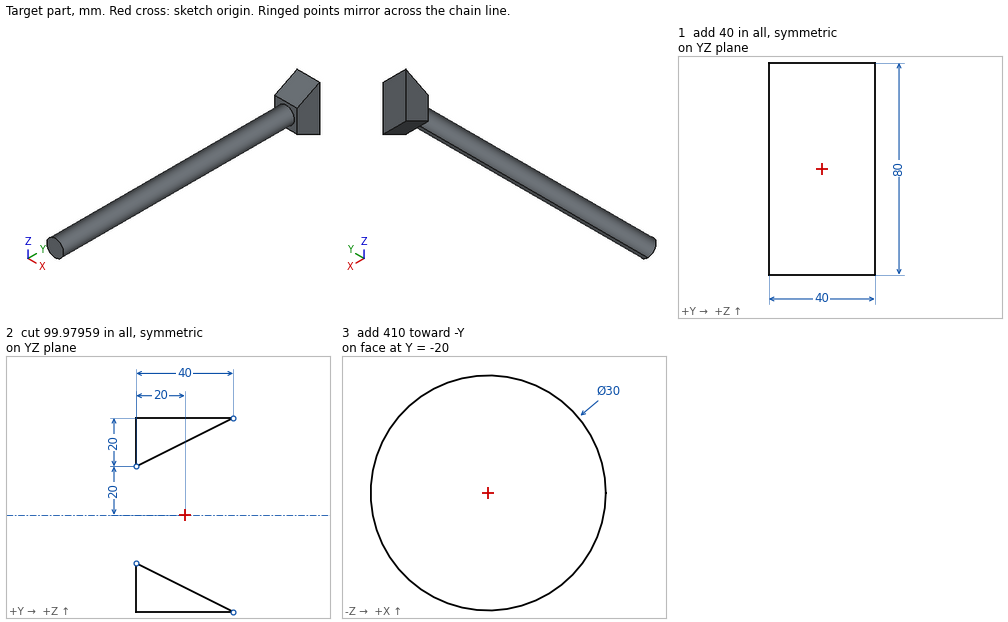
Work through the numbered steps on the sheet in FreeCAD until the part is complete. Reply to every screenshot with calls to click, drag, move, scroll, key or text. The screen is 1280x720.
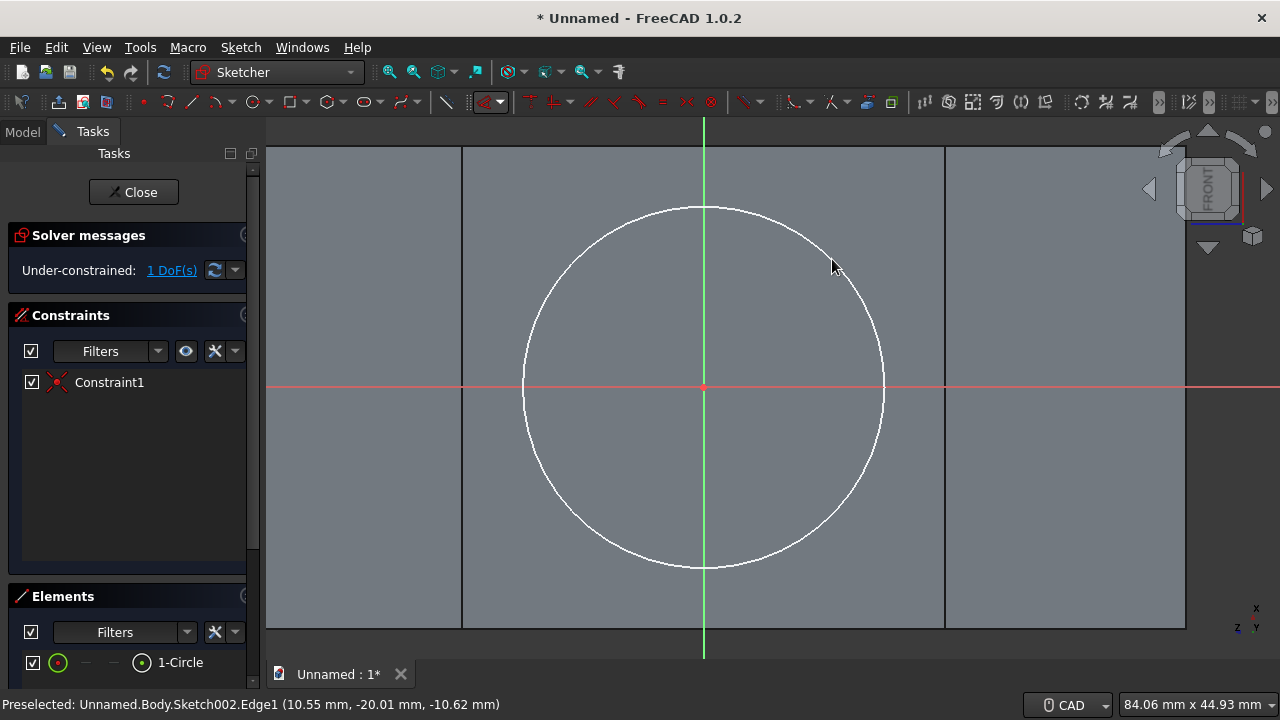
click(831, 259)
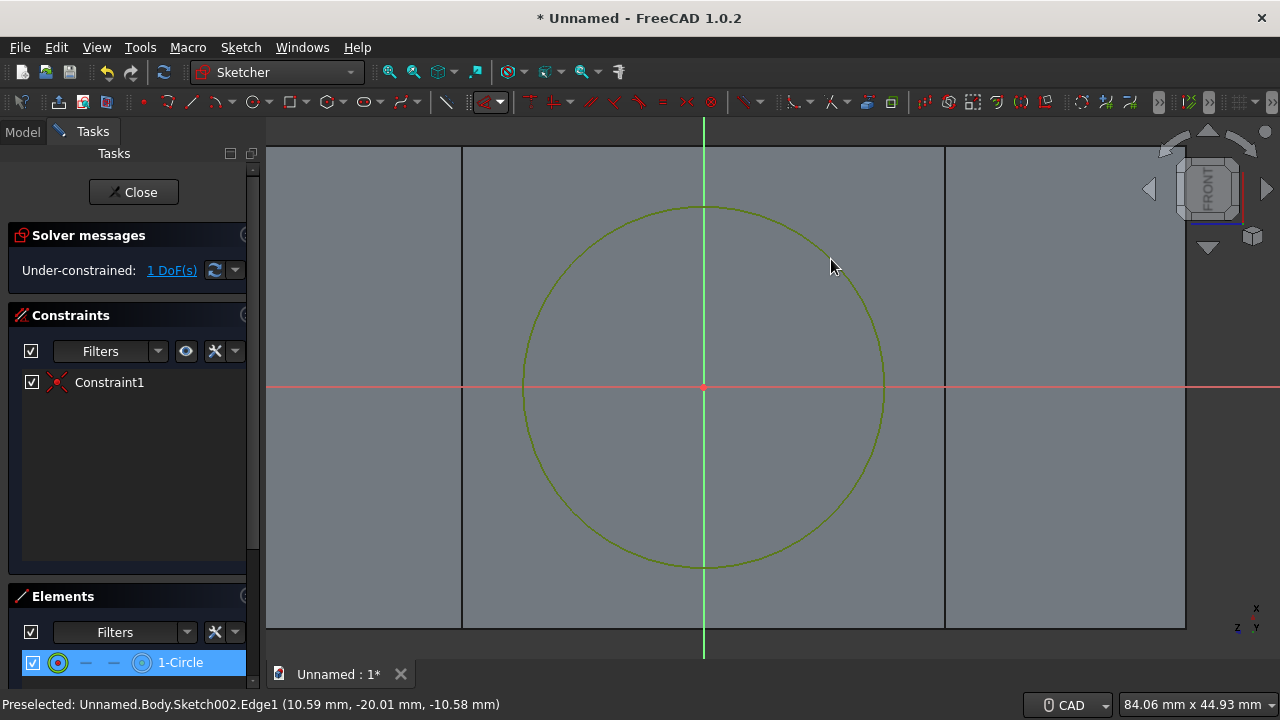
key(k)
key(o)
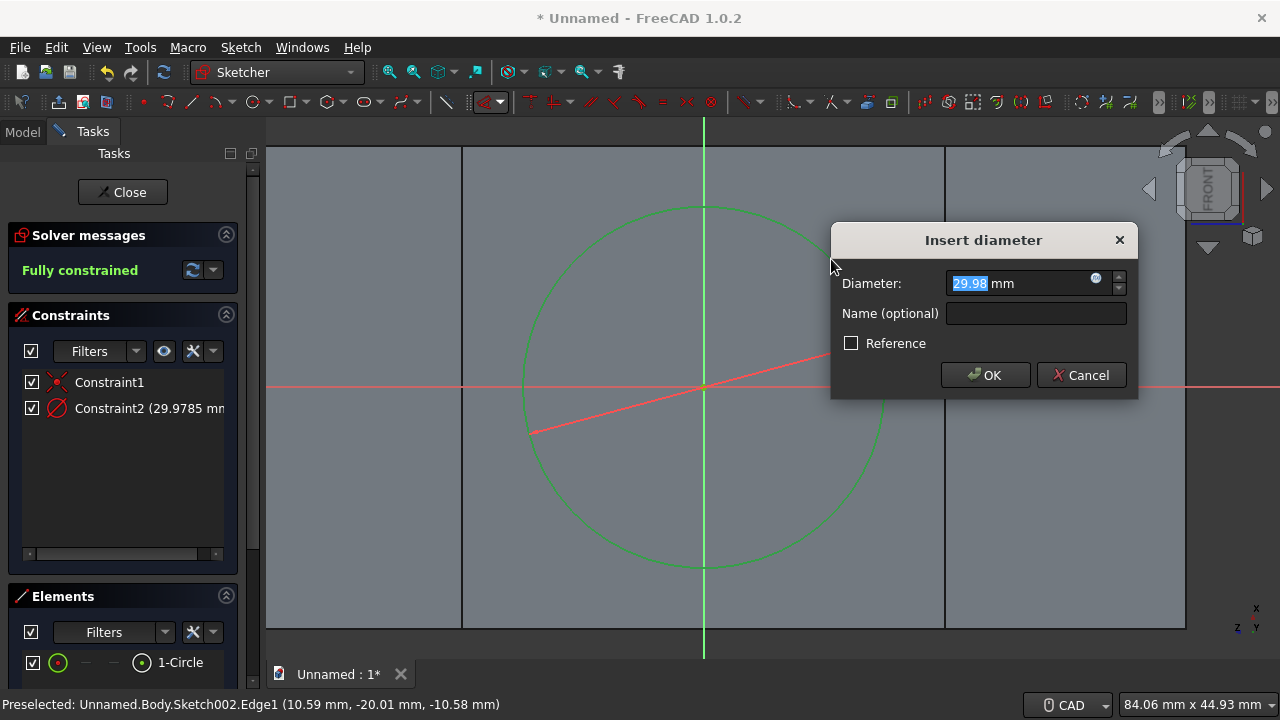
text(30)
key(Return)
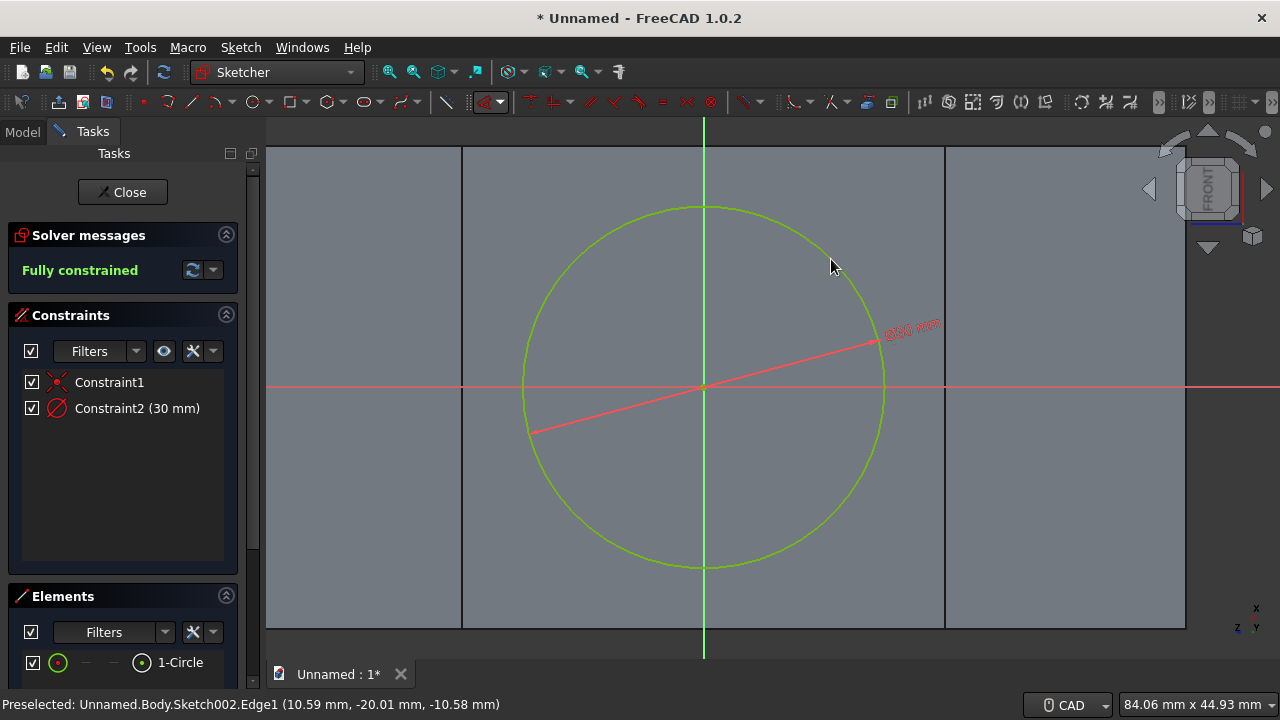
click(123, 192)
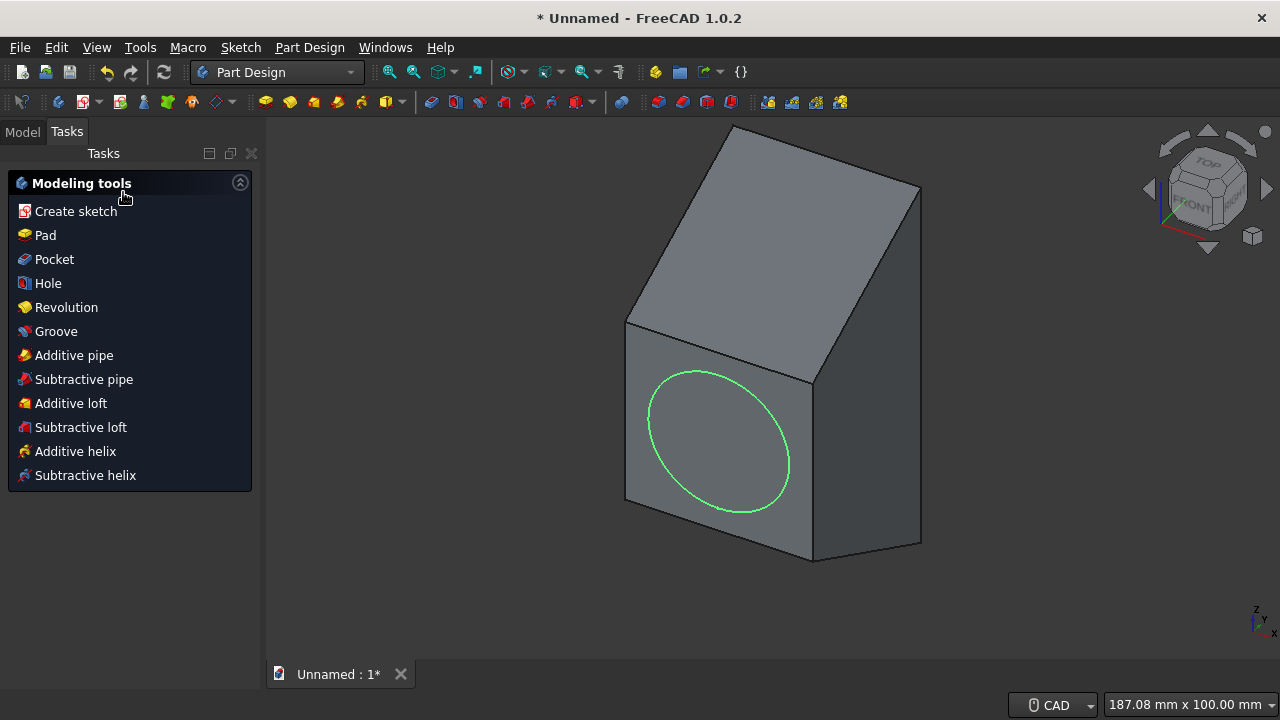
click(266, 102)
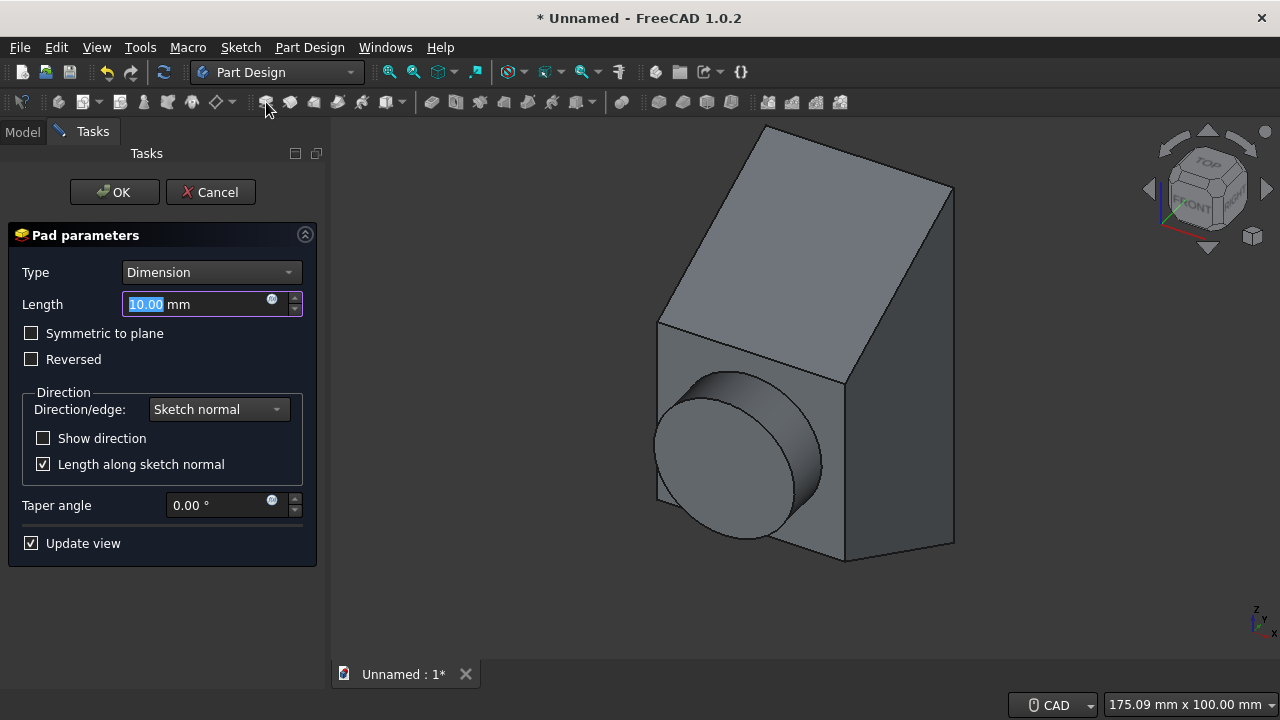
text(410)
key(Tab)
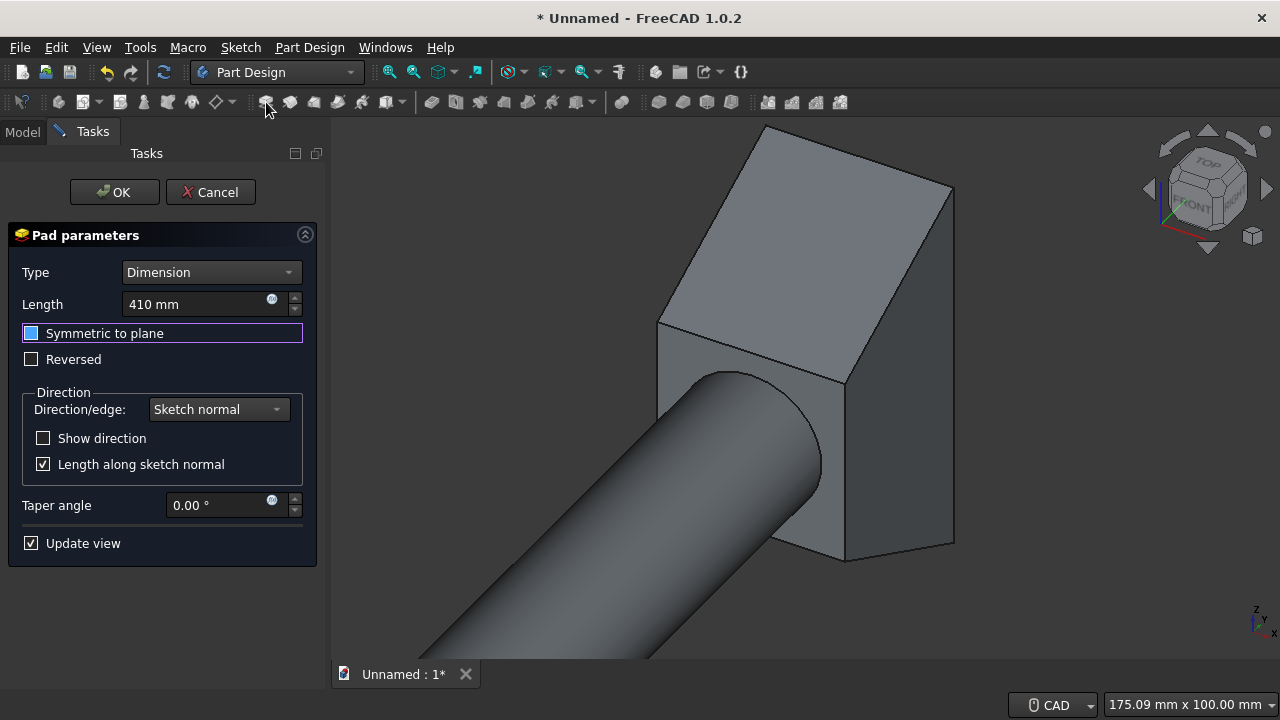
click(115, 192)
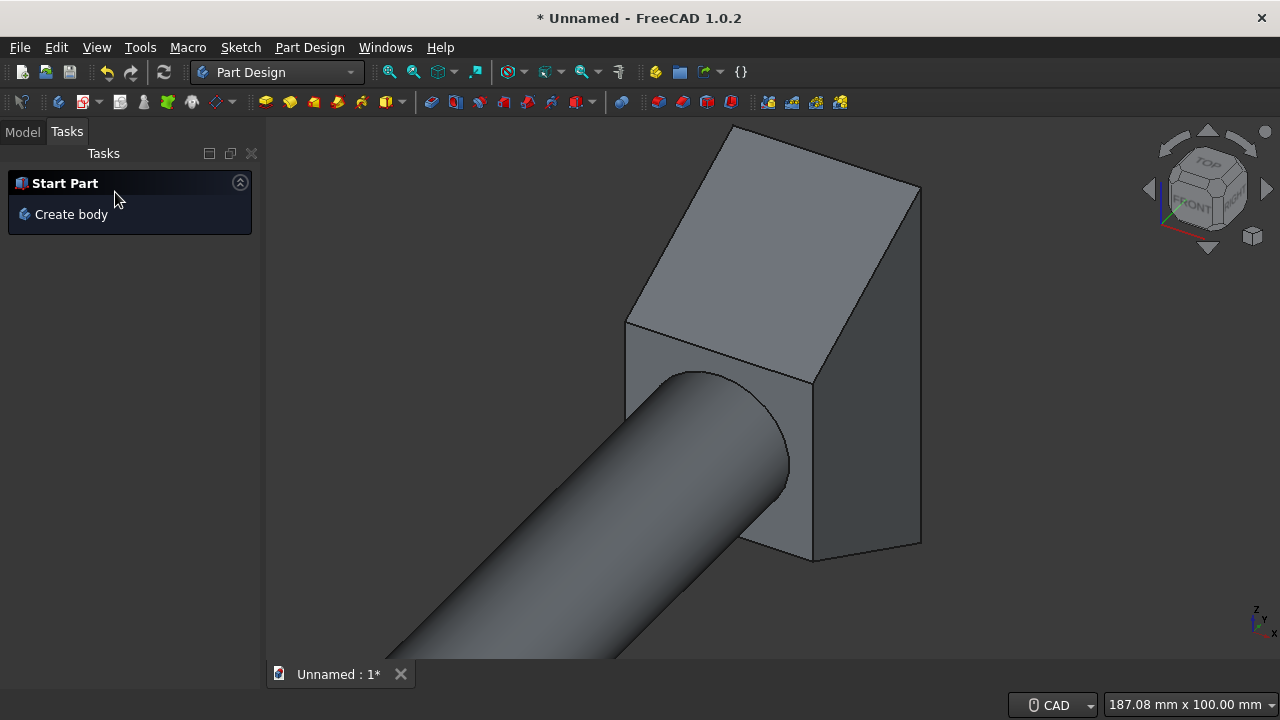
key(0)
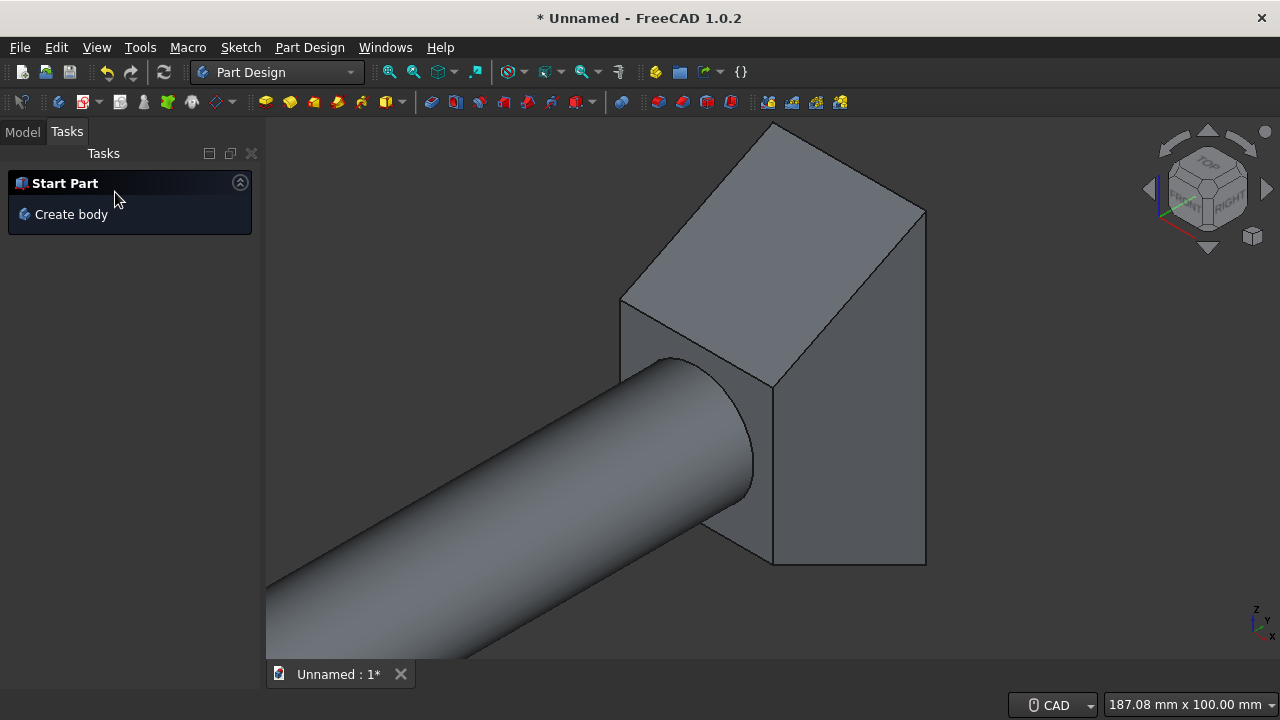
key(v)
key(f)